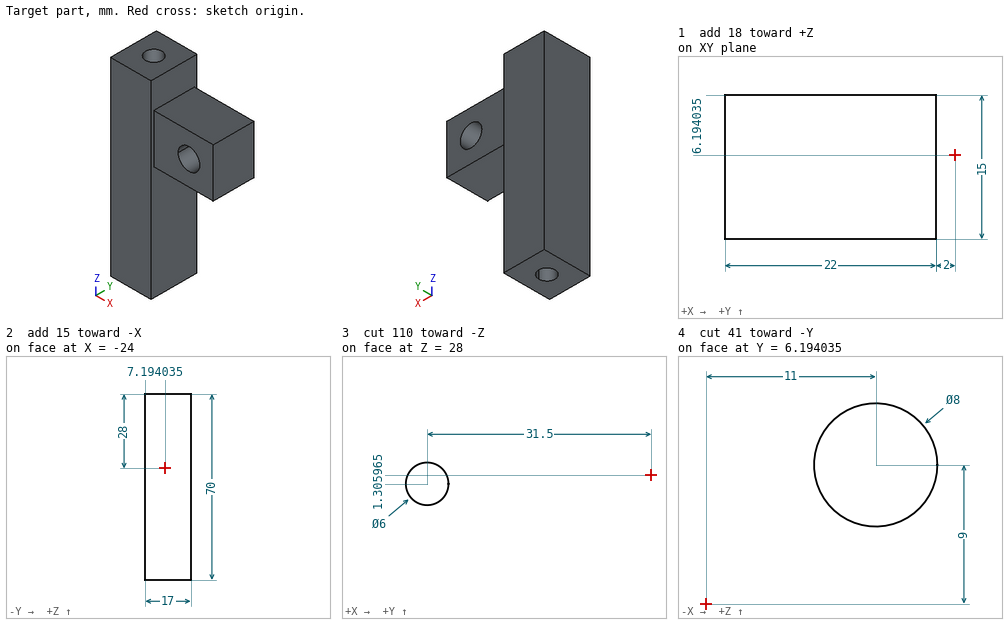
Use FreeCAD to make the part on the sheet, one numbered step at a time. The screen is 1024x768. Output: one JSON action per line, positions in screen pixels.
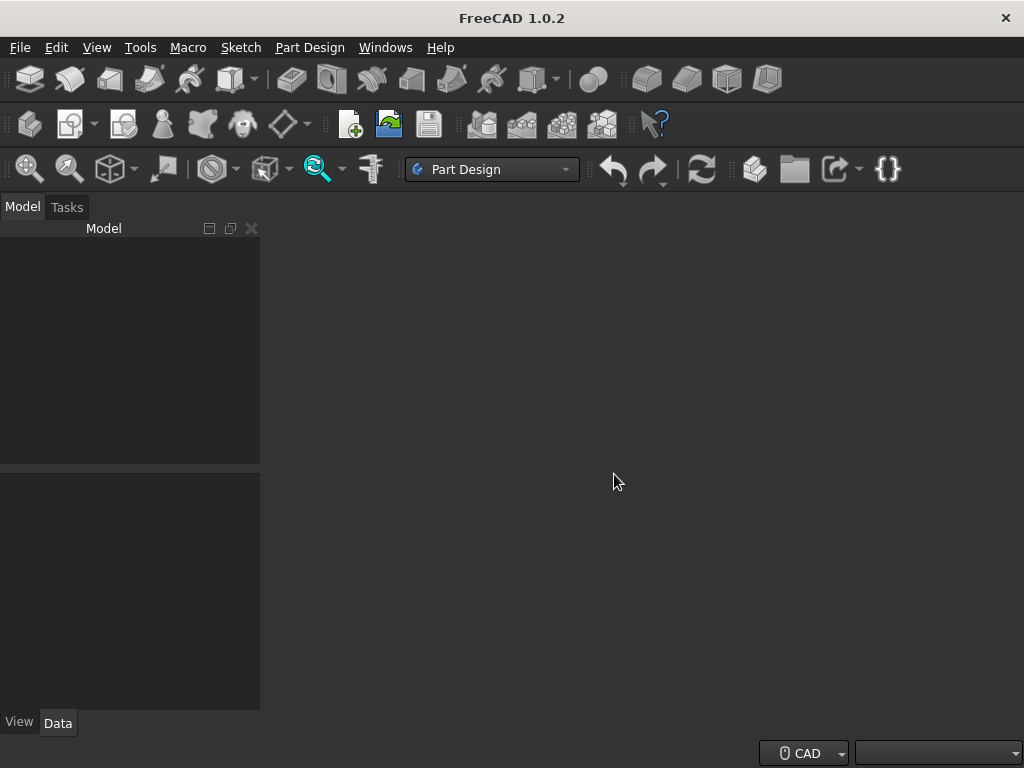
{"action": "left_click", "coordinate": [350, 124]}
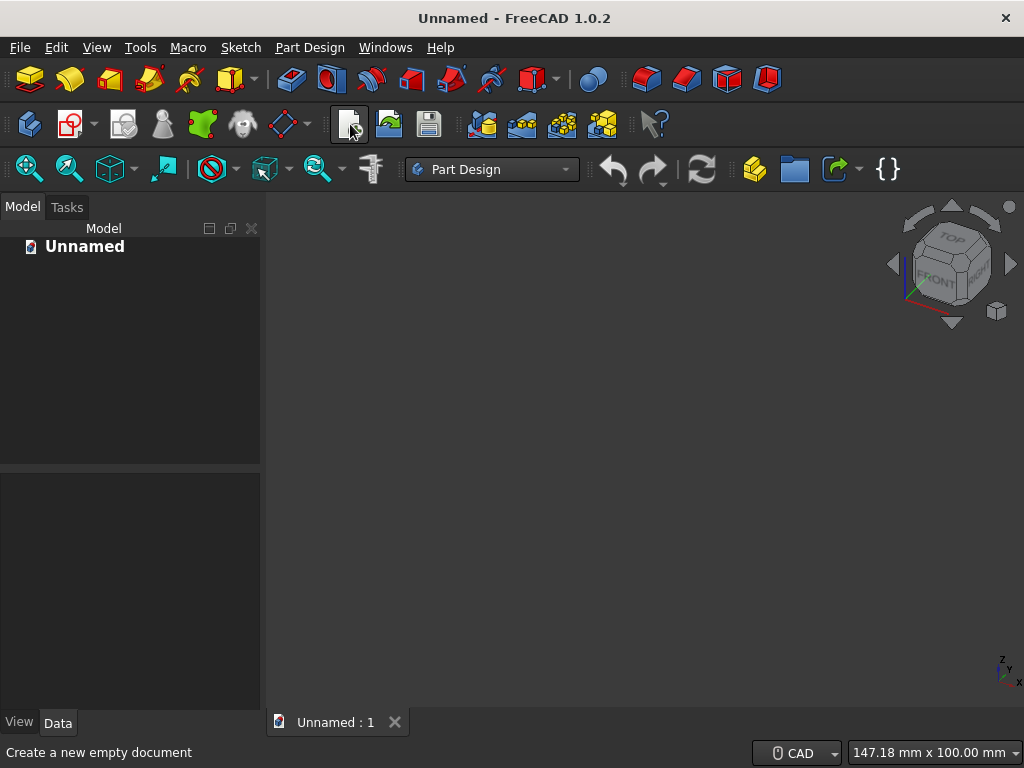
{"action": "left_click", "coordinate": [70, 124]}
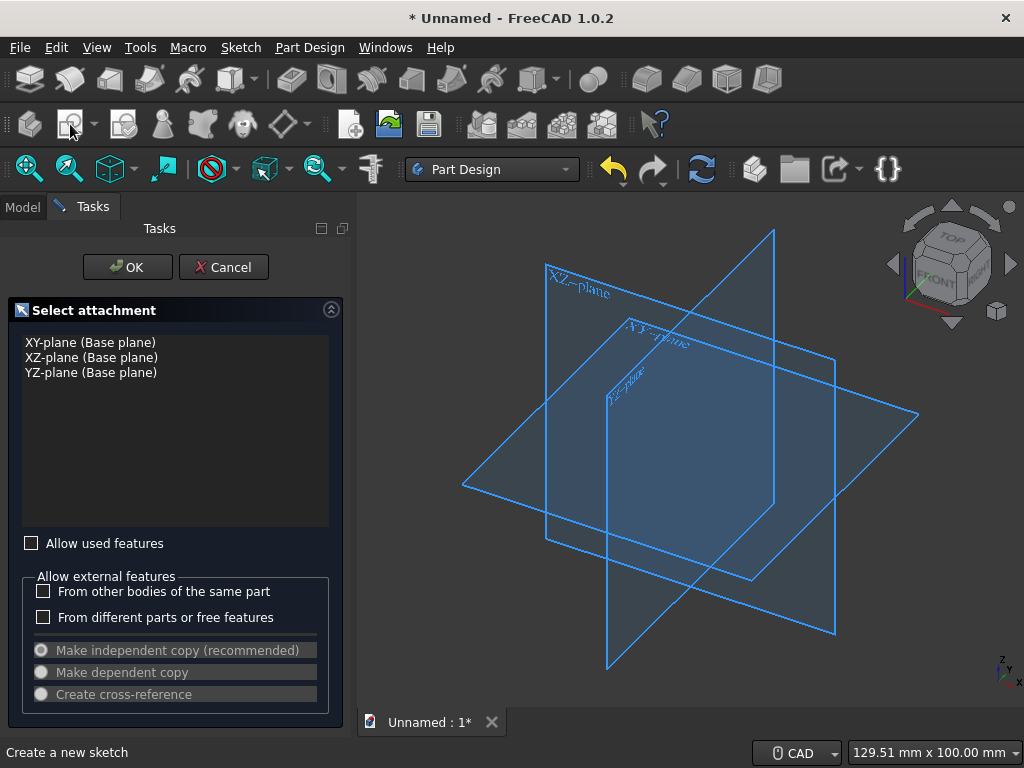
{"action": "left_click", "coordinate": [82, 342]}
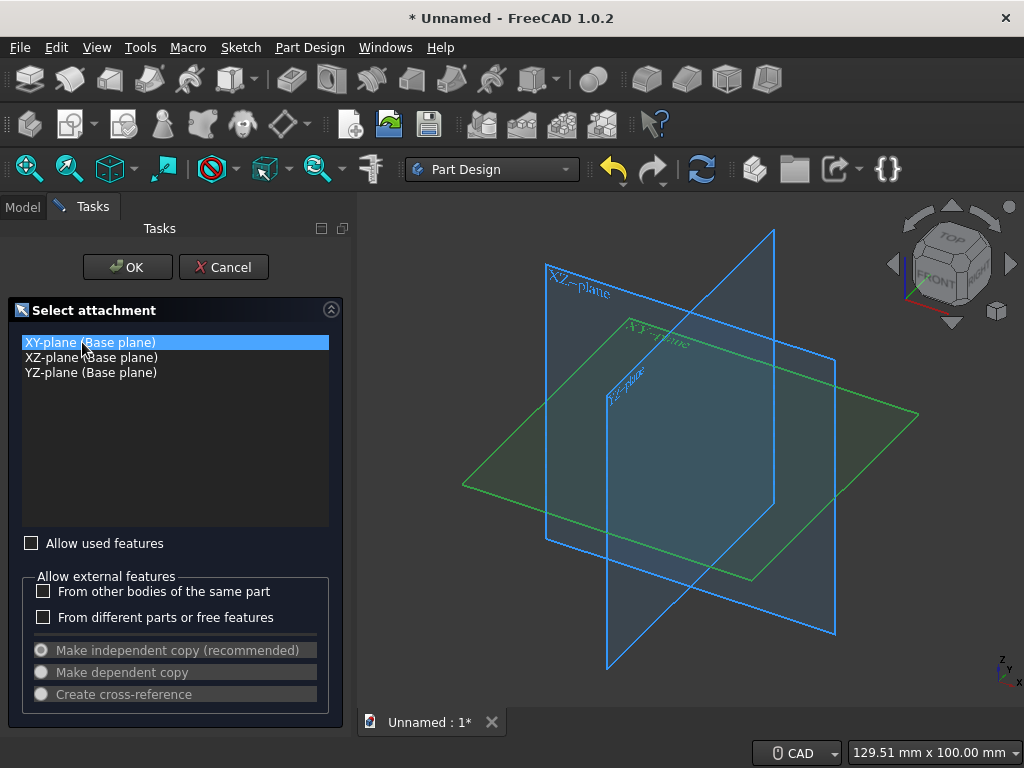
{"action": "left_click", "coordinate": [128, 267]}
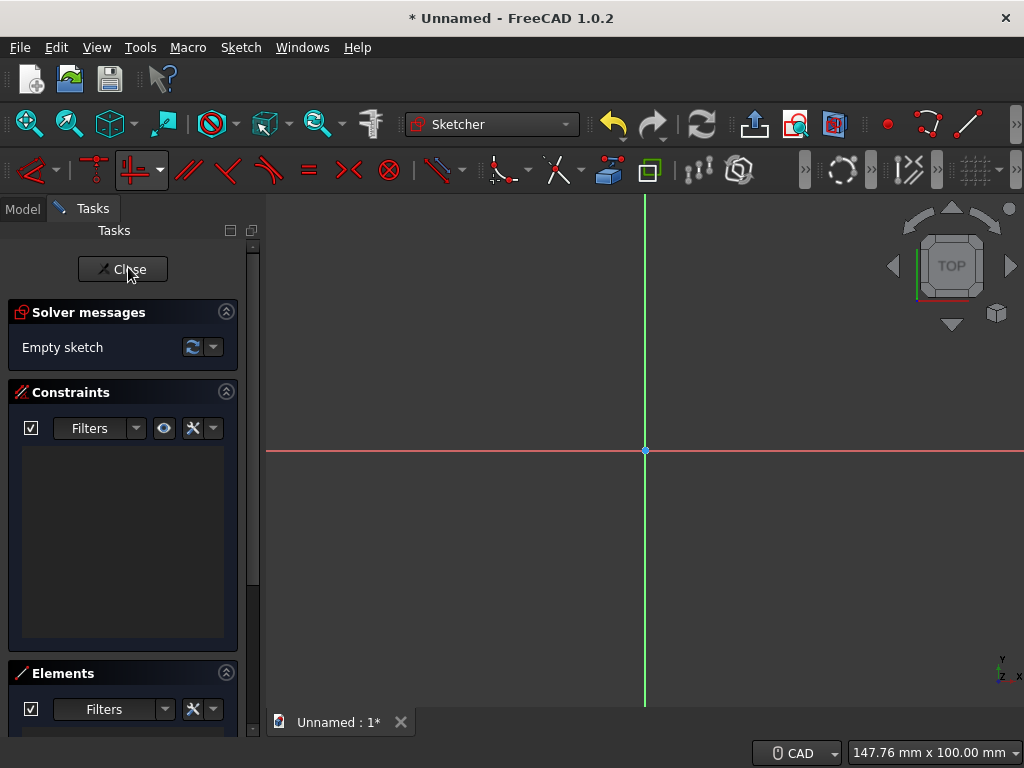
{"action": "scroll", "coordinate": [586, 460], "scroll_direction": "up", "scroll_amount": 6}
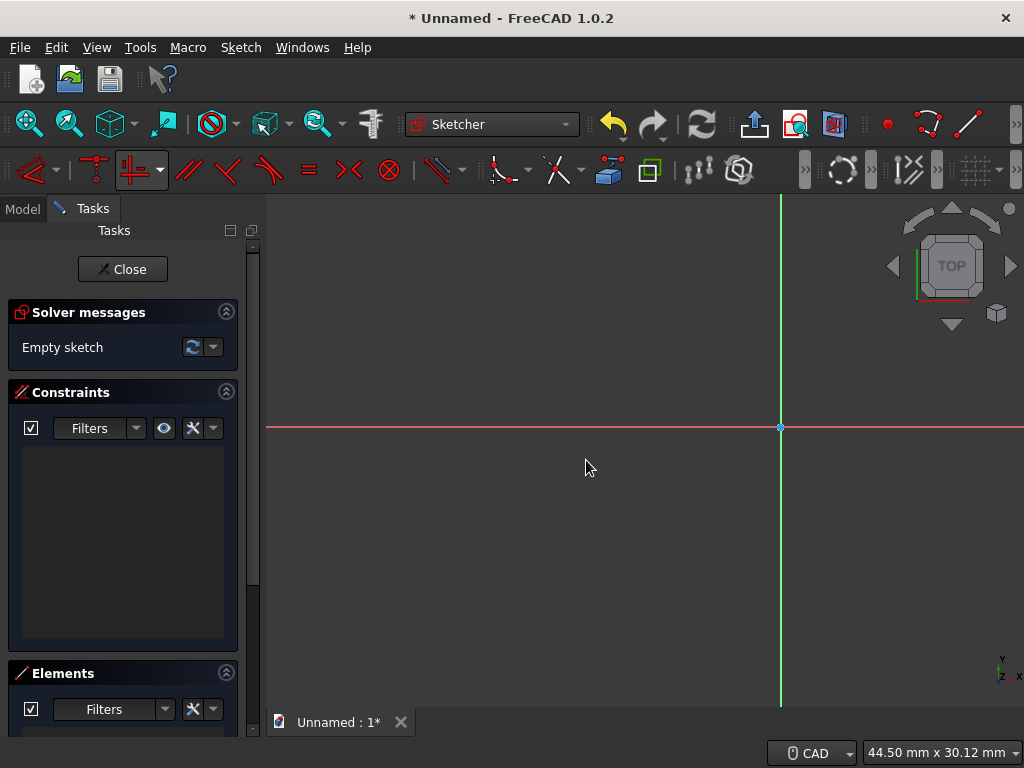
{"action": "key", "text": "g r"}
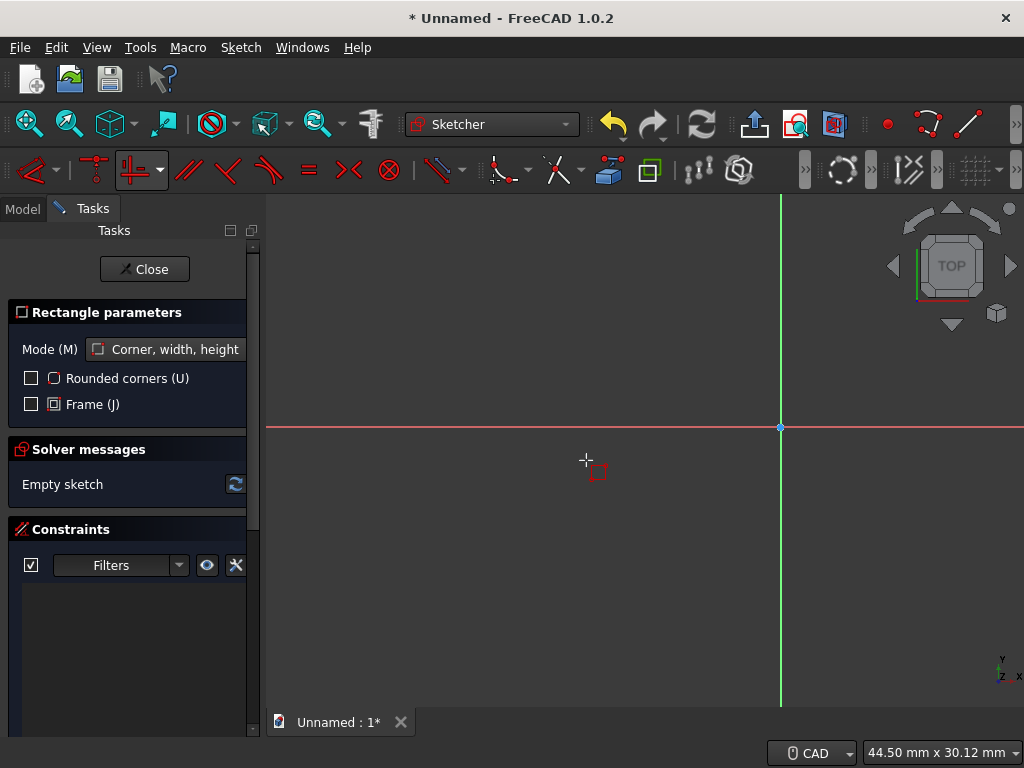
{"action": "left_click", "coordinate": [372, 322]}
{"action": "mouse_move", "coordinate": [747, 577]}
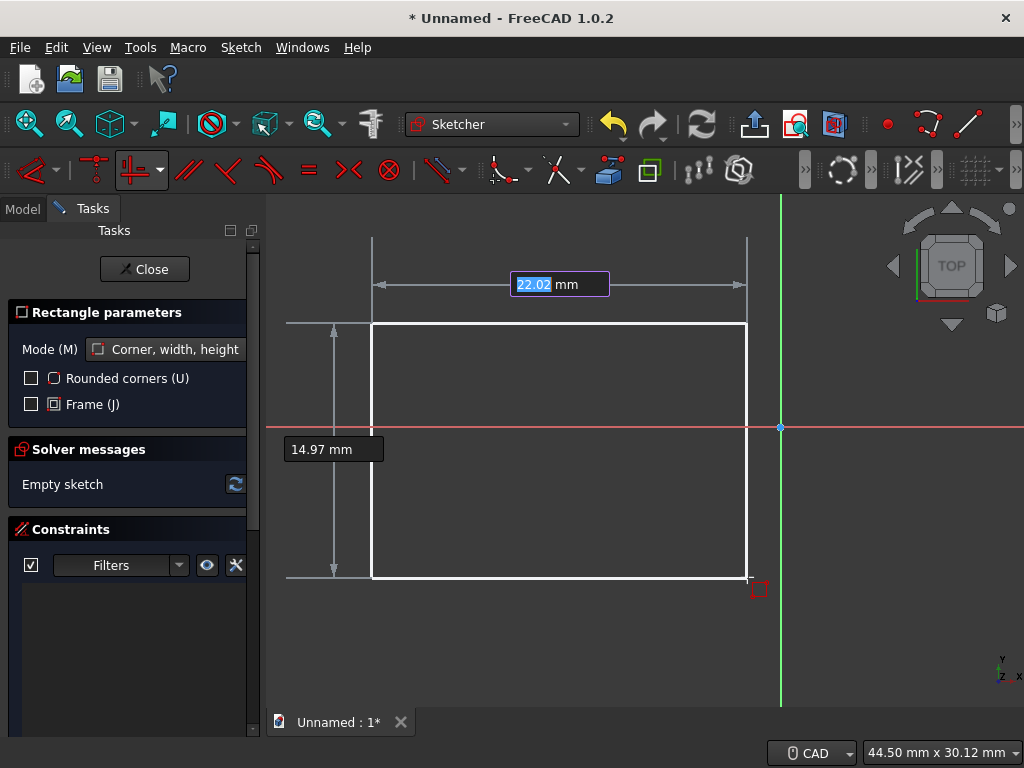
{"action": "type", "text": "22"}
{"action": "key", "text": "Tab"}
{"action": "type", "text": "15"}
{"action": "key", "text": "Return"}
{"action": "key", "text": "Escape"}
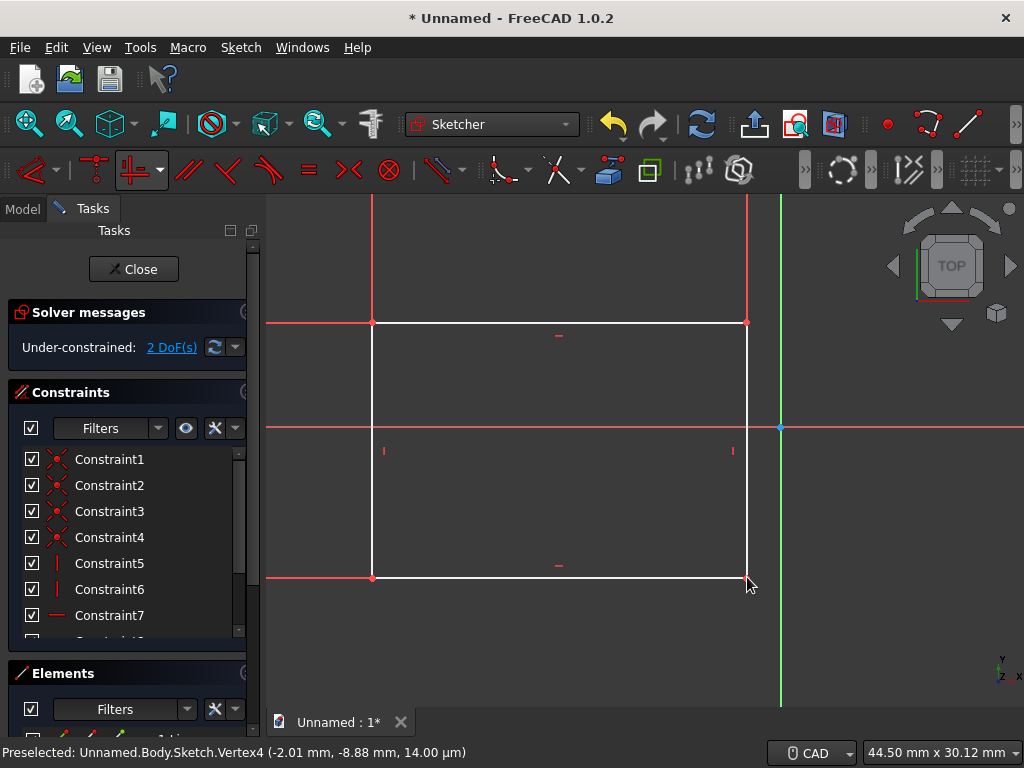
{"action": "left_click", "coordinate": [32, 170]}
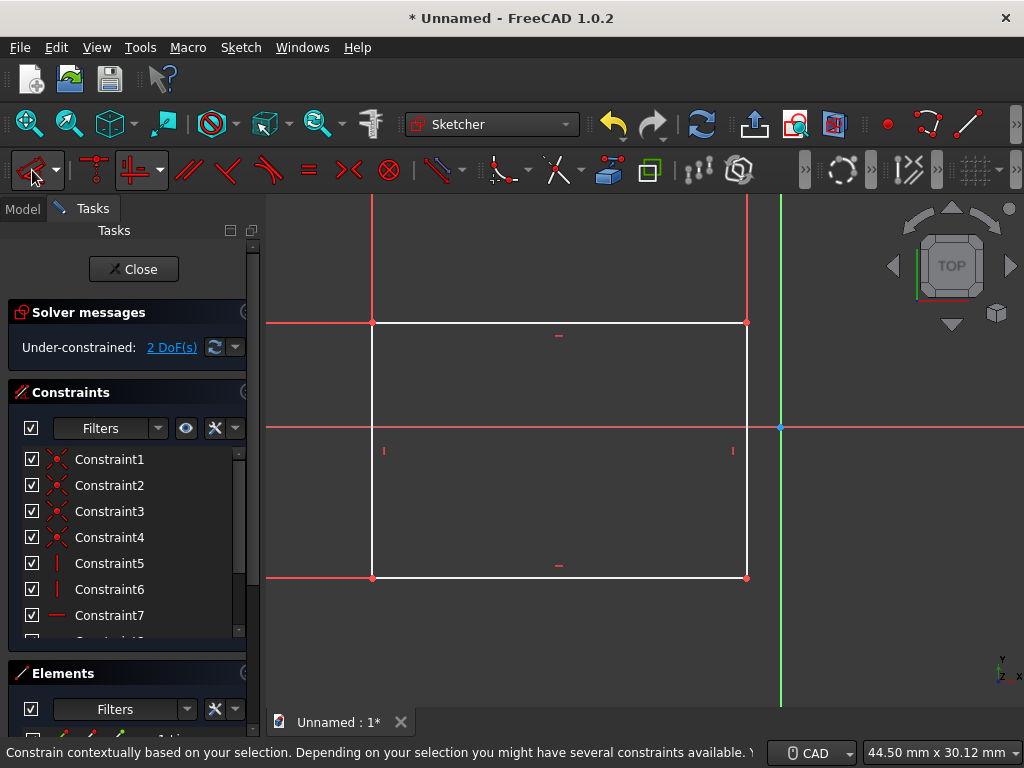
{"action": "left_click", "coordinate": [747, 578]}
{"action": "left_click", "coordinate": [764, 612]}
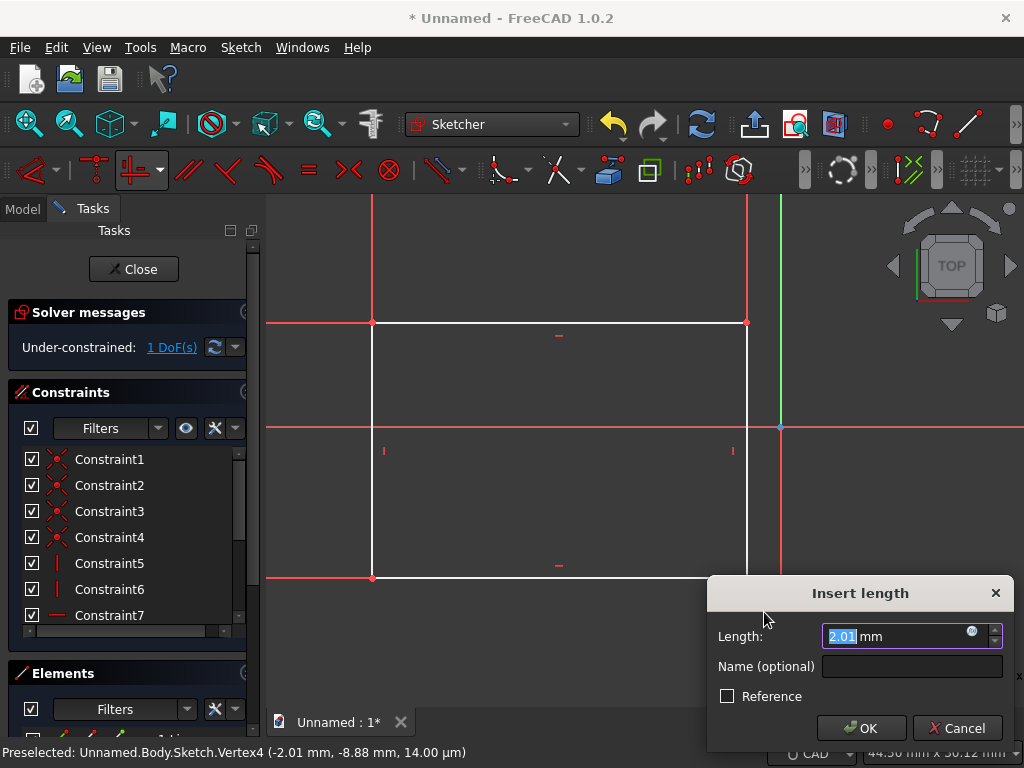
{"action": "type", "text": "2"}
{"action": "key", "text": "Return"}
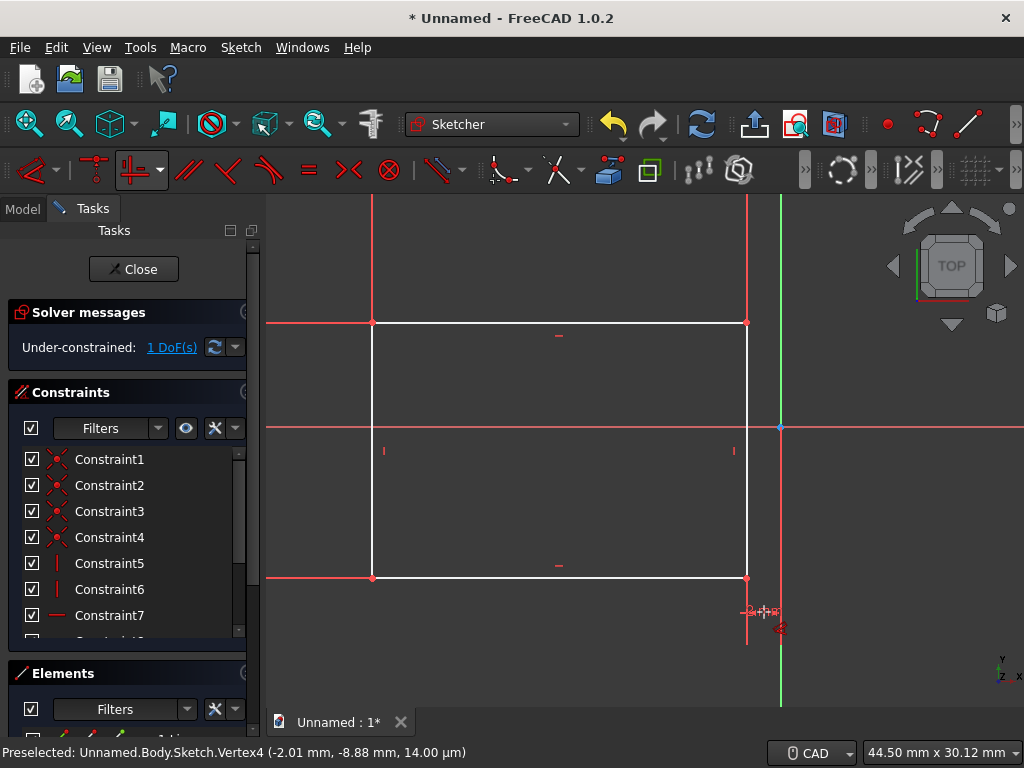
{"action": "left_click", "coordinate": [372, 323]}
{"action": "left_click", "coordinate": [815, 375]}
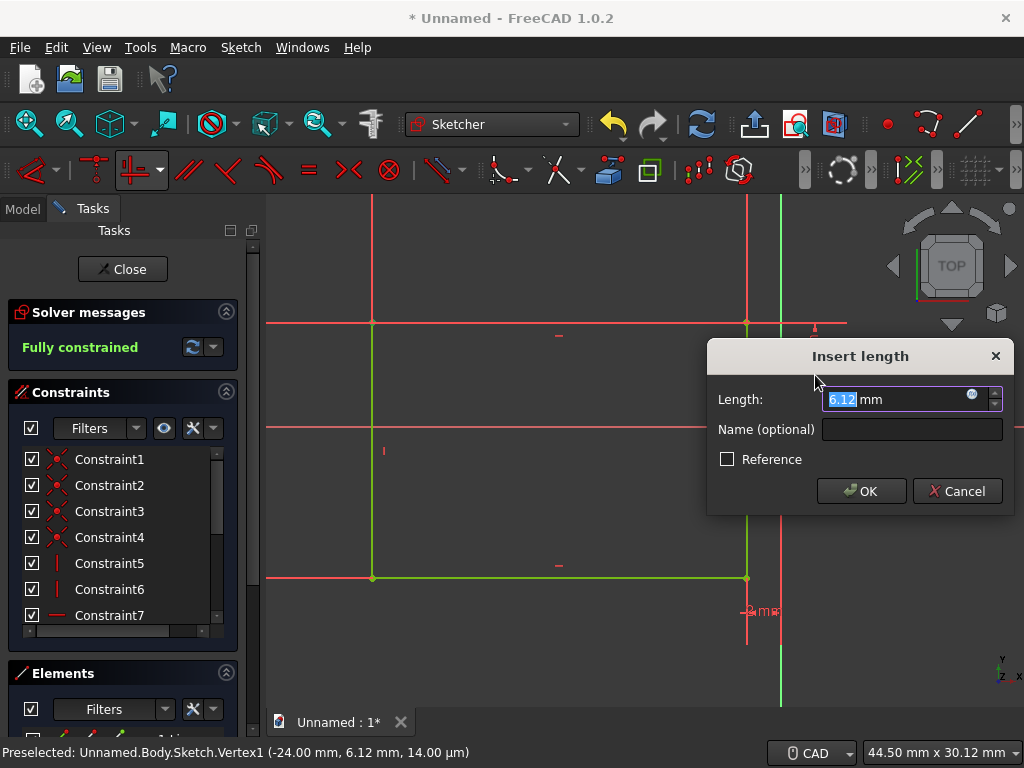
{"action": "type", "text": "6.194035"}
{"action": "key", "text": "Return"}
{"action": "key", "text": "Escape"}